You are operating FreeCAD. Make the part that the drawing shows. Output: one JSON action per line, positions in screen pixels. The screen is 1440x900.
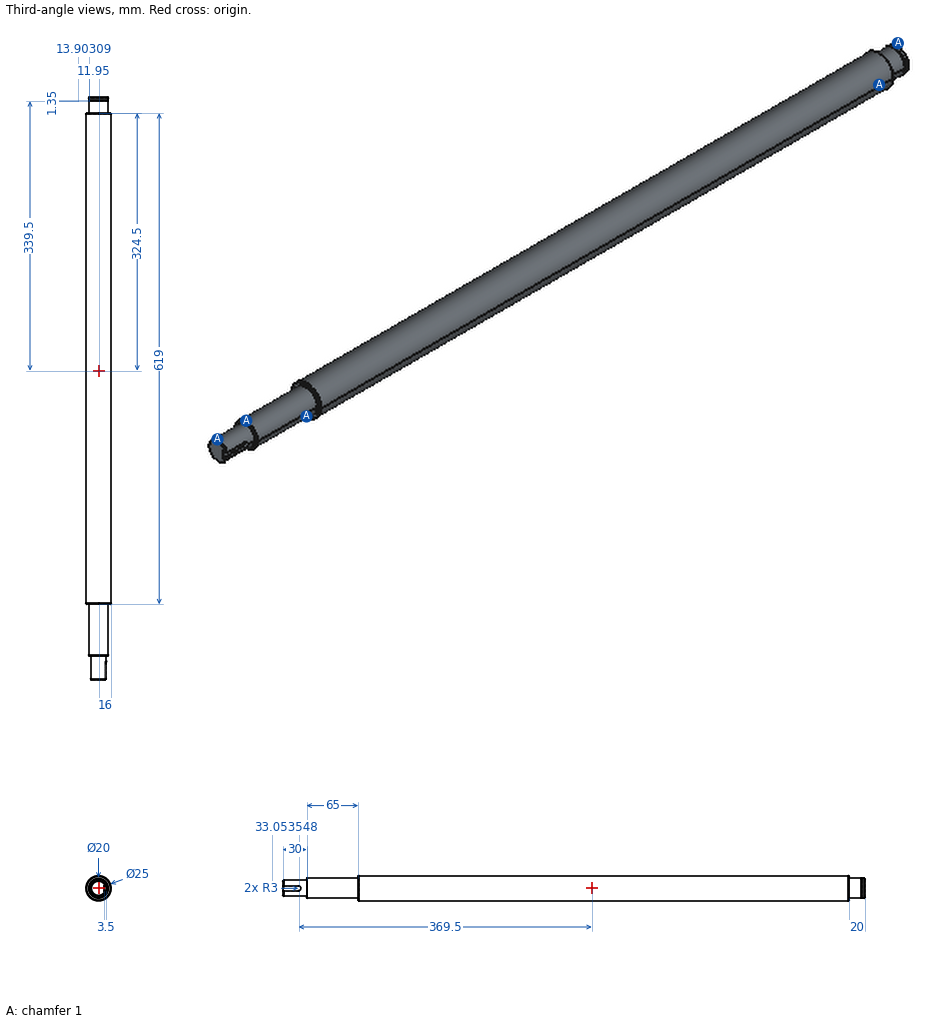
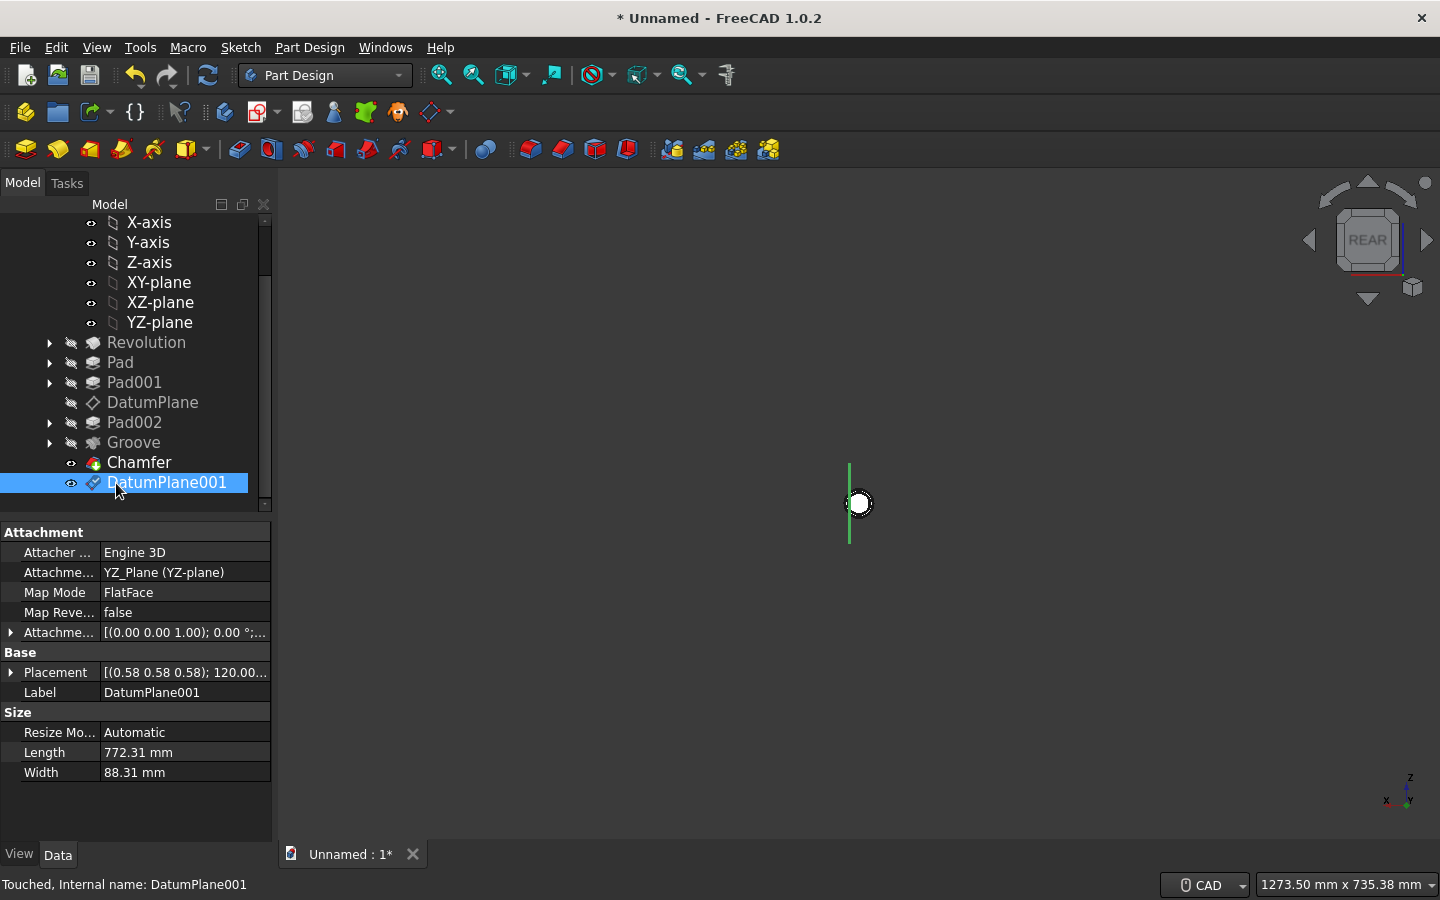
{"action": "left_click", "coordinate": [258, 112]}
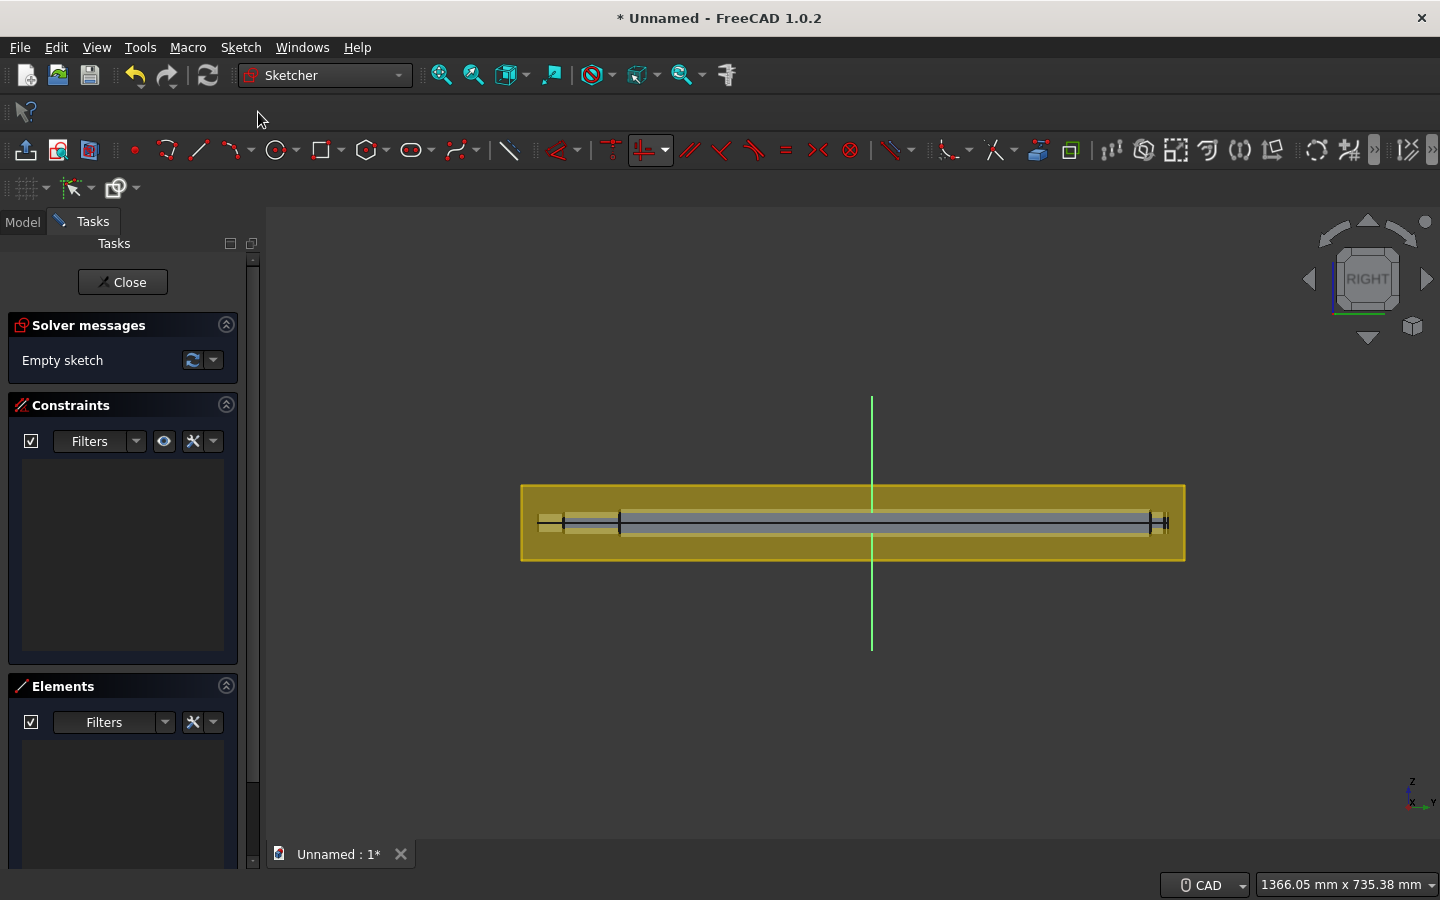
{"action": "left_click", "coordinate": [90, 150]}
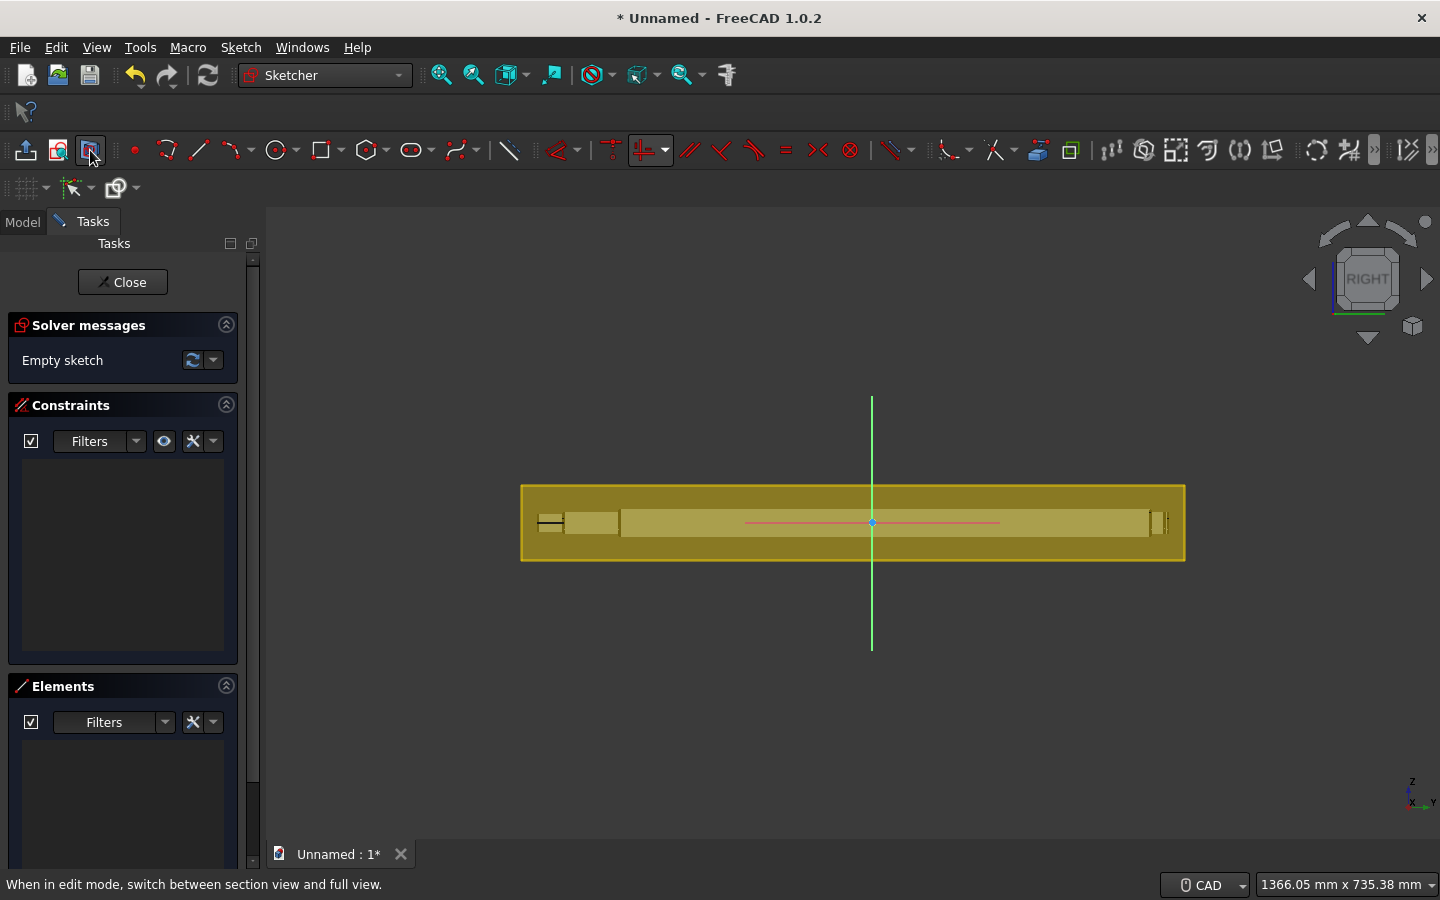
{"action": "scroll", "coordinate": [528, 523], "scroll_direction": "up", "scroll_amount": 15}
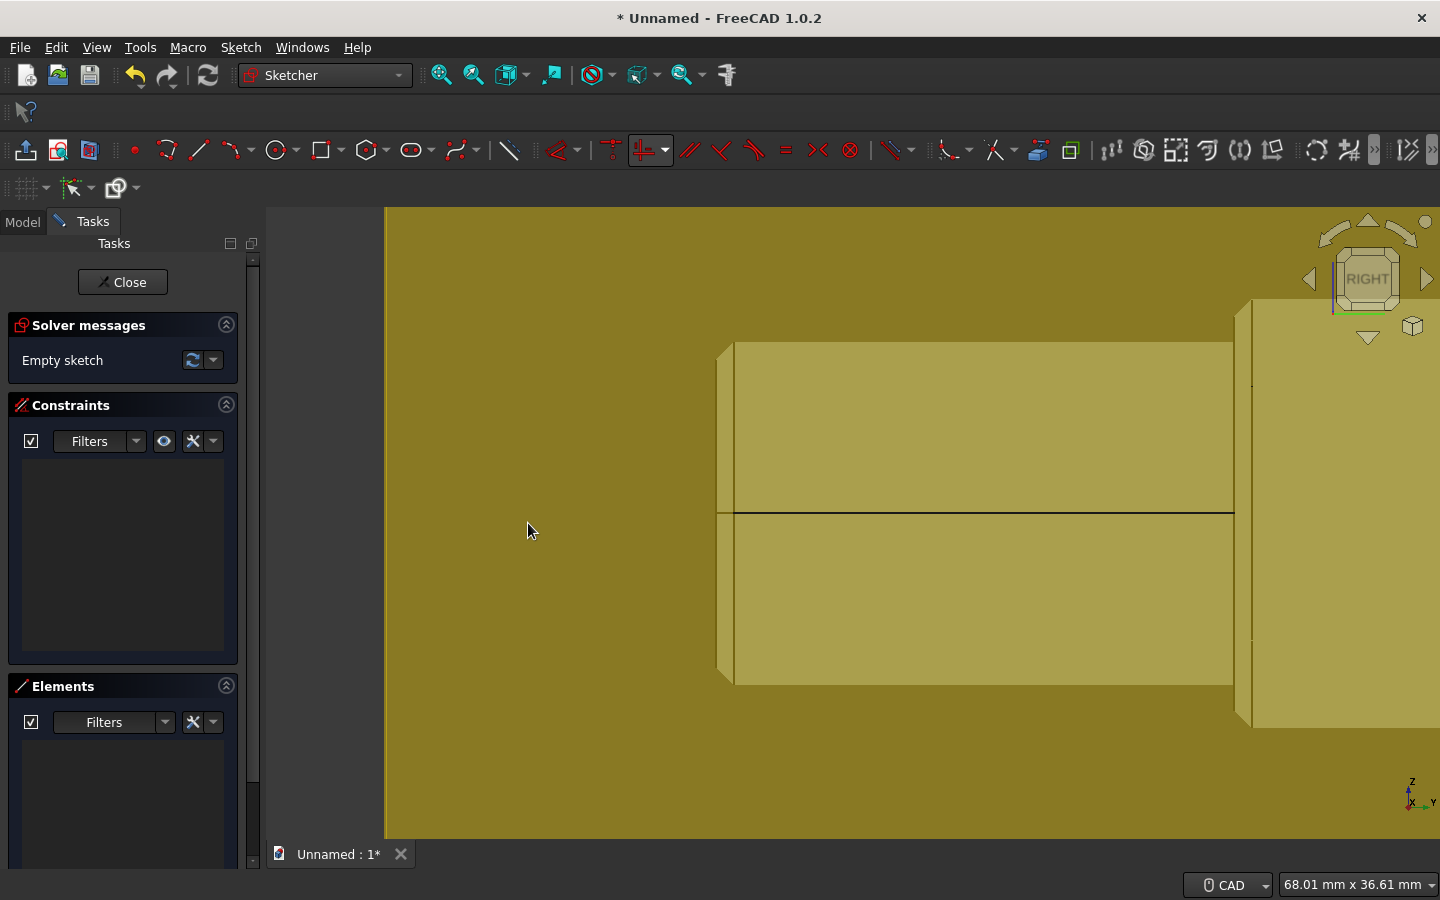
{"action": "left_click", "coordinate": [412, 150]}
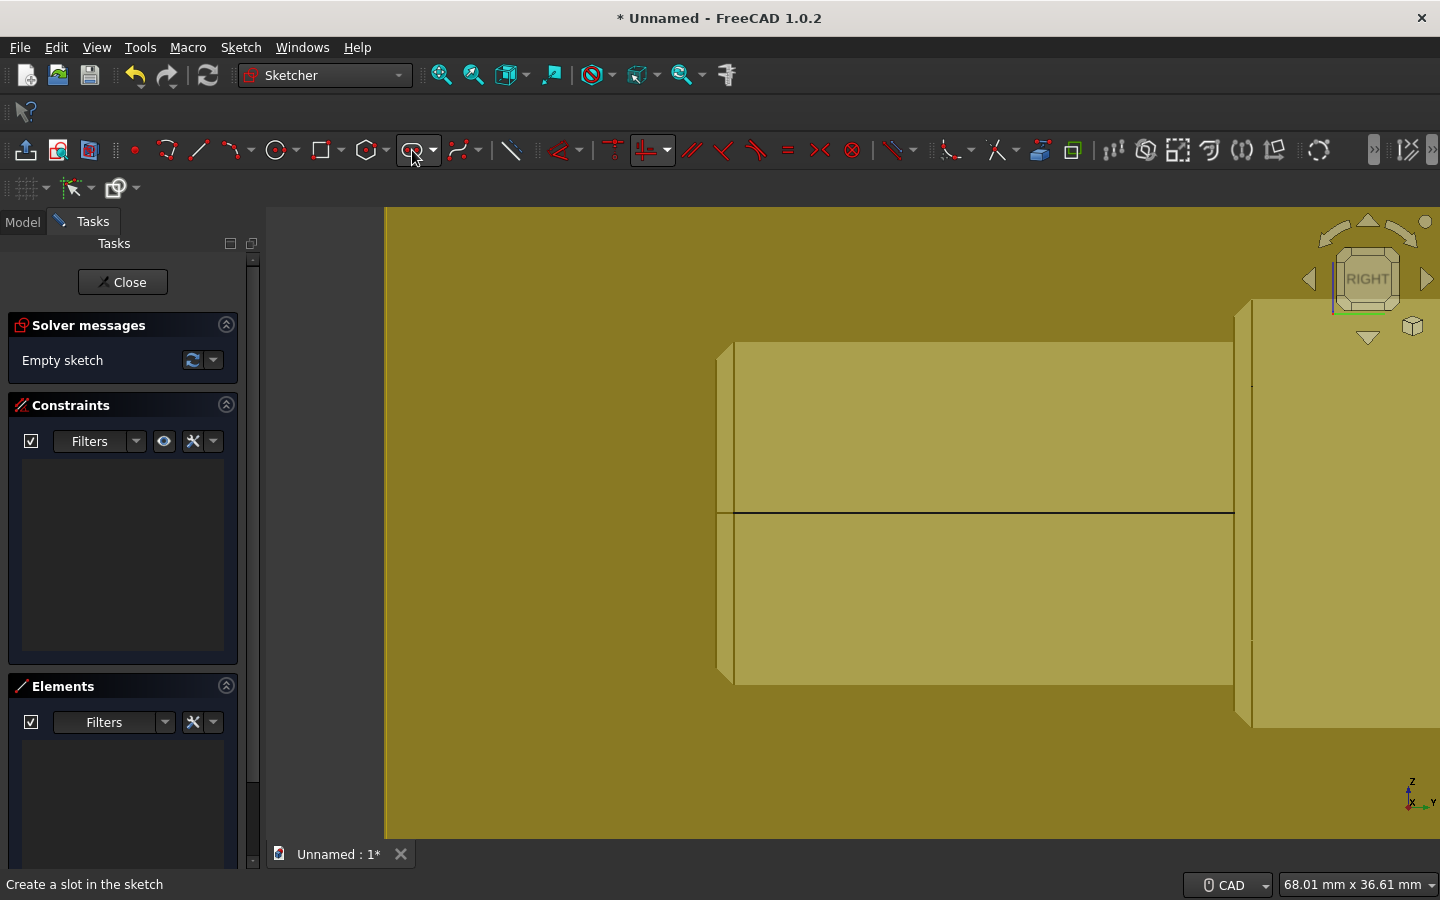
{"action": "left_click", "coordinate": [491, 513]}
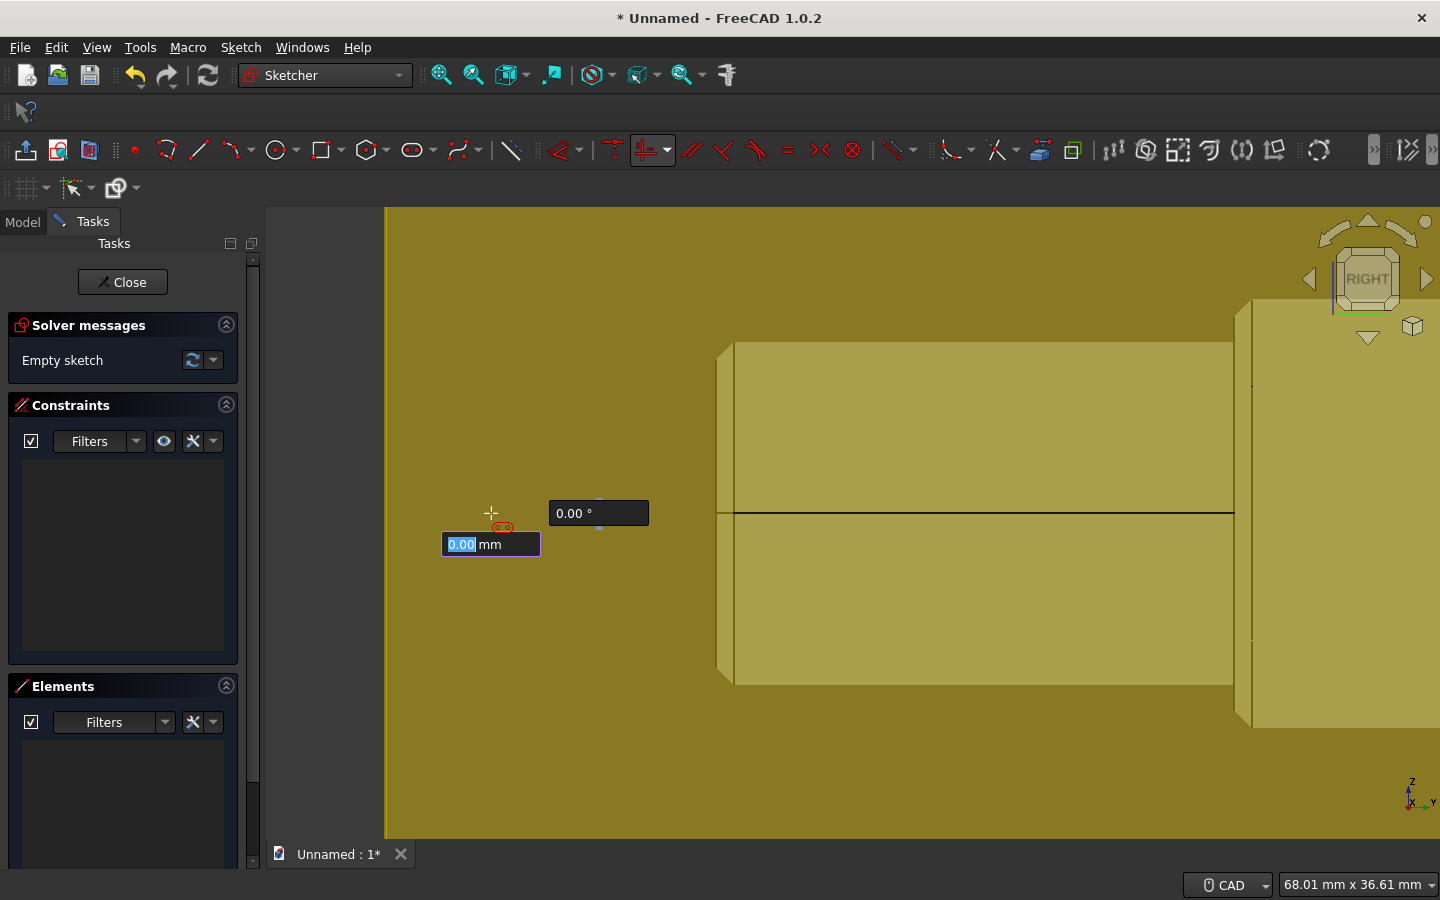
{"action": "left_click", "coordinate": [1062, 504]}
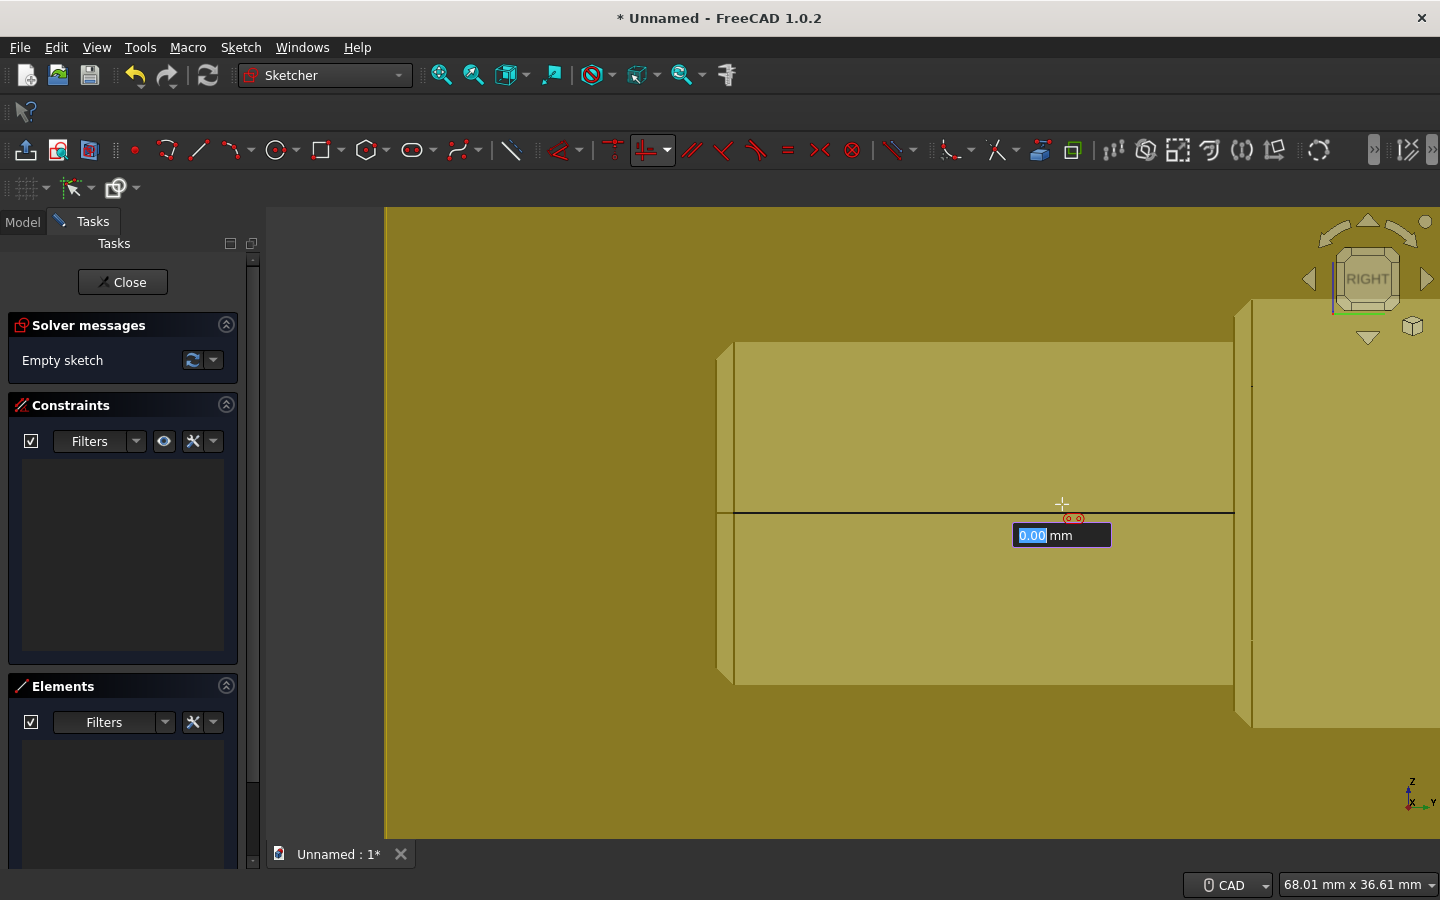
{"action": "left_click", "coordinate": [776, 565]}
{"action": "key", "text": "Escape"}